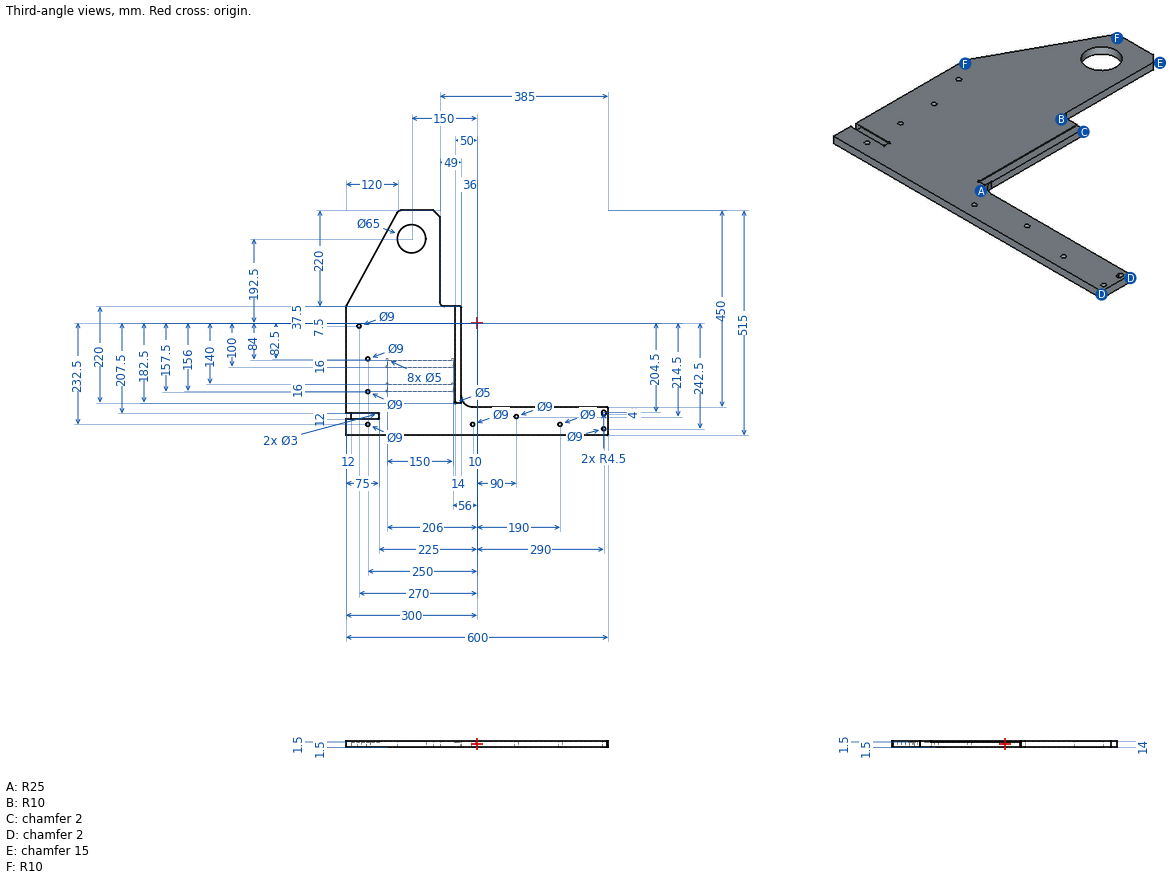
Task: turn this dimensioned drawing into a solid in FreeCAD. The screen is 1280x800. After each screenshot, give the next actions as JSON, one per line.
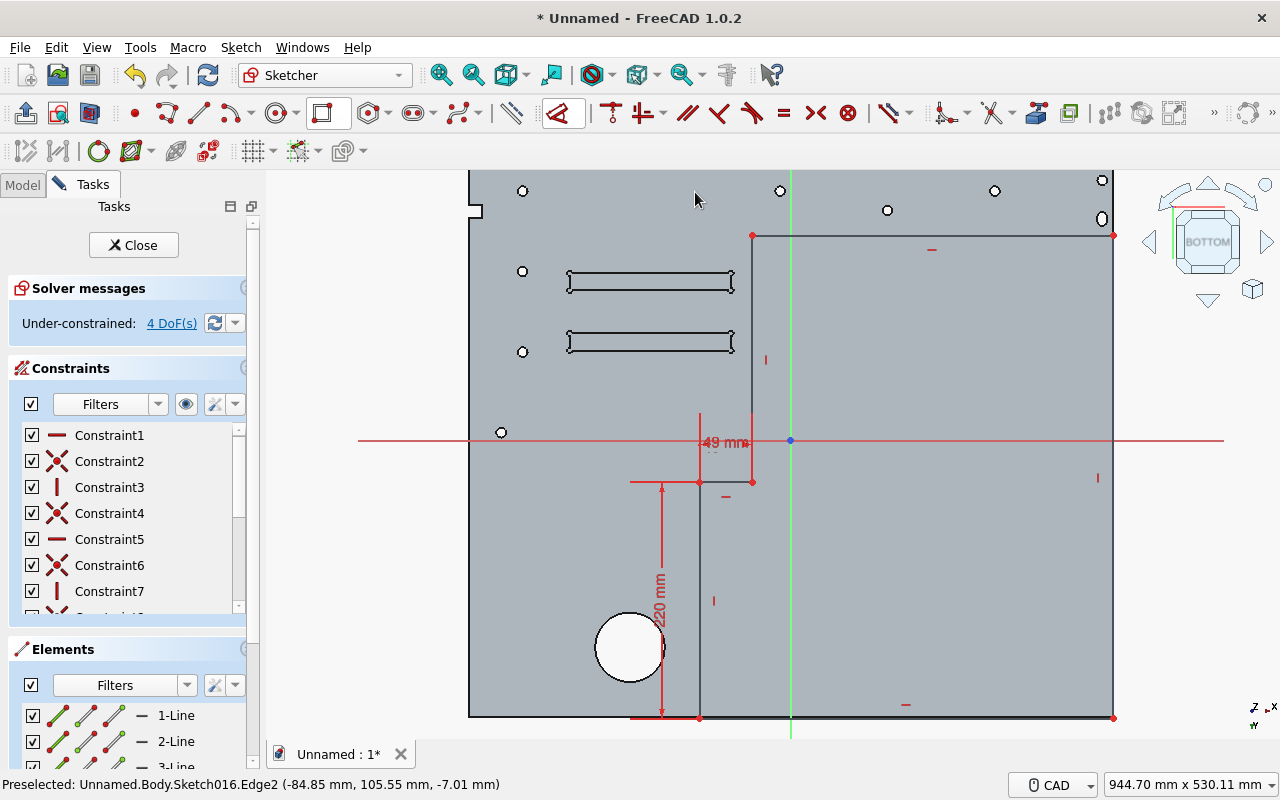
{"action": "scroll", "coordinate": [294, 359], "scroll_direction": "down", "scroll_amount": 1}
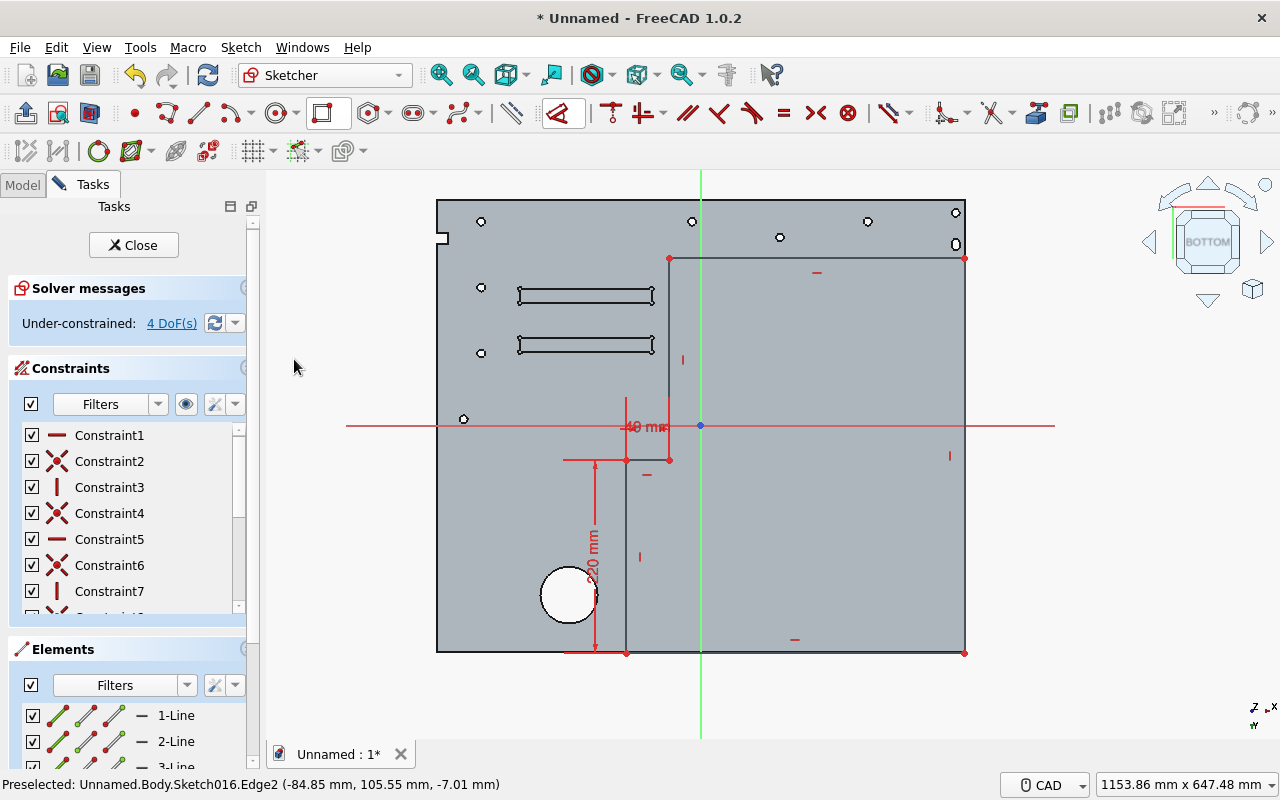
{"action": "left_click", "coordinate": [728, 653]}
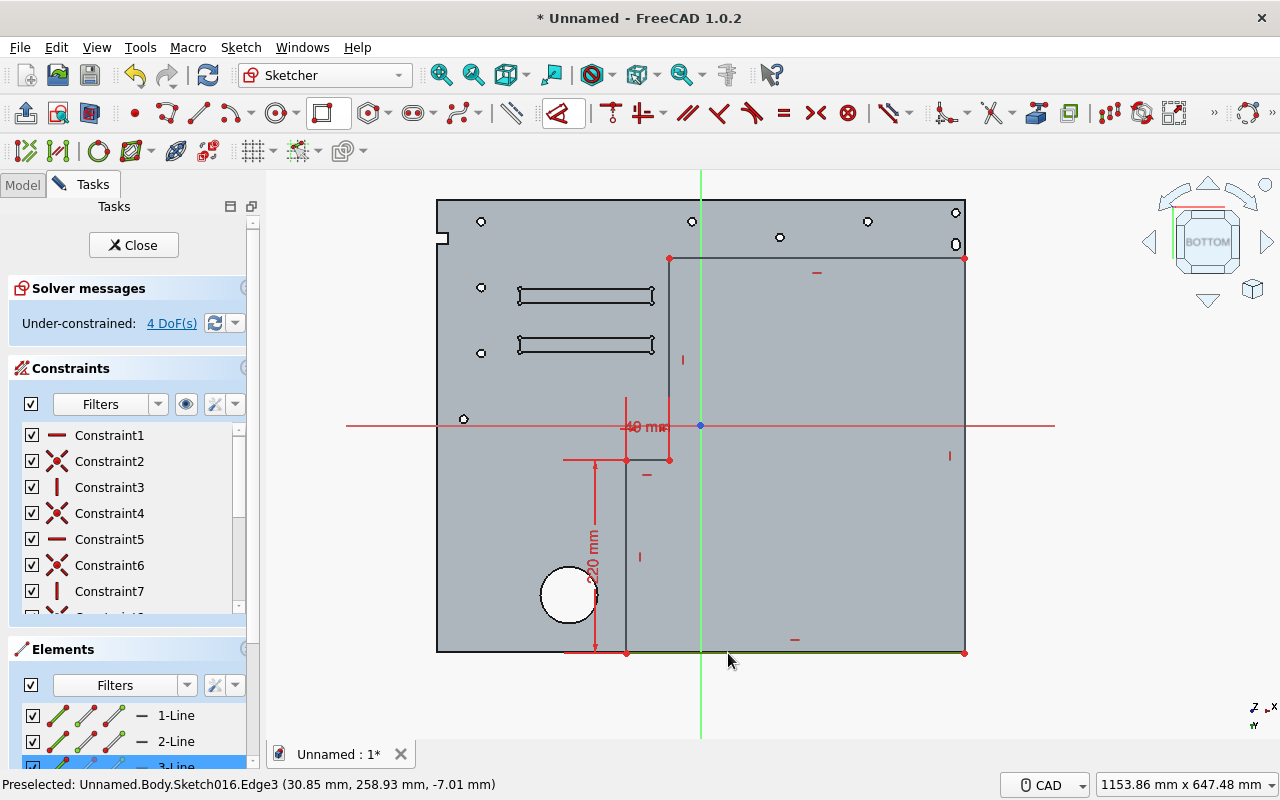
{"action": "left_click", "coordinate": [580, 114]}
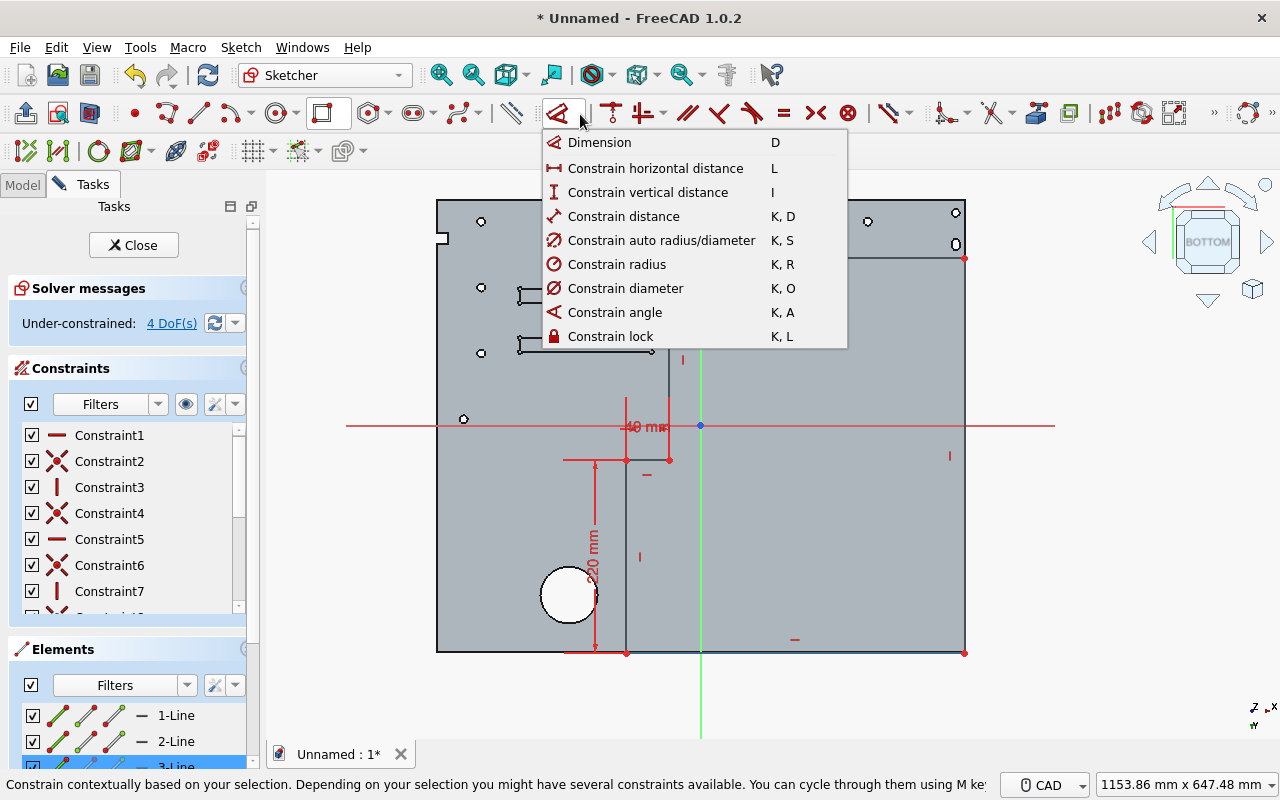
{"action": "left_click", "coordinate": [695, 168]}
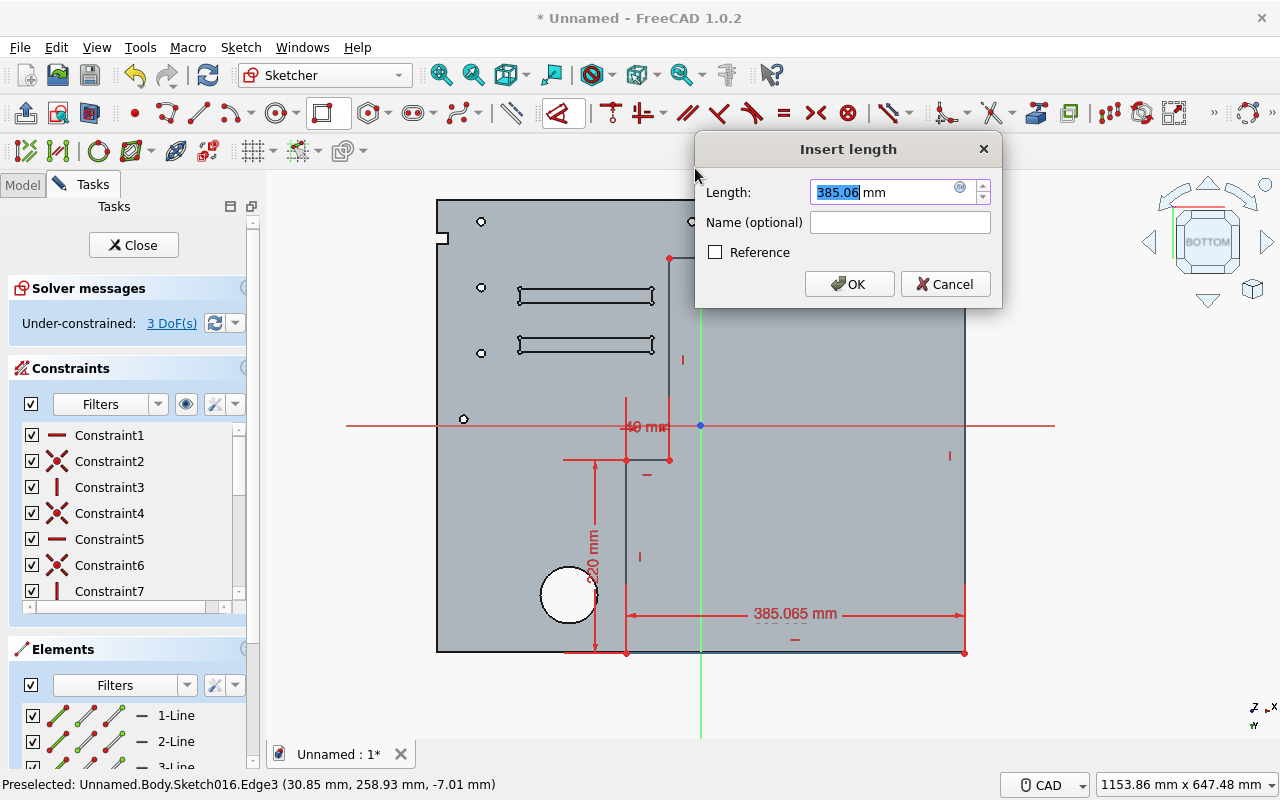
{"action": "type", "text": "385"}
{"action": "key", "text": "Return"}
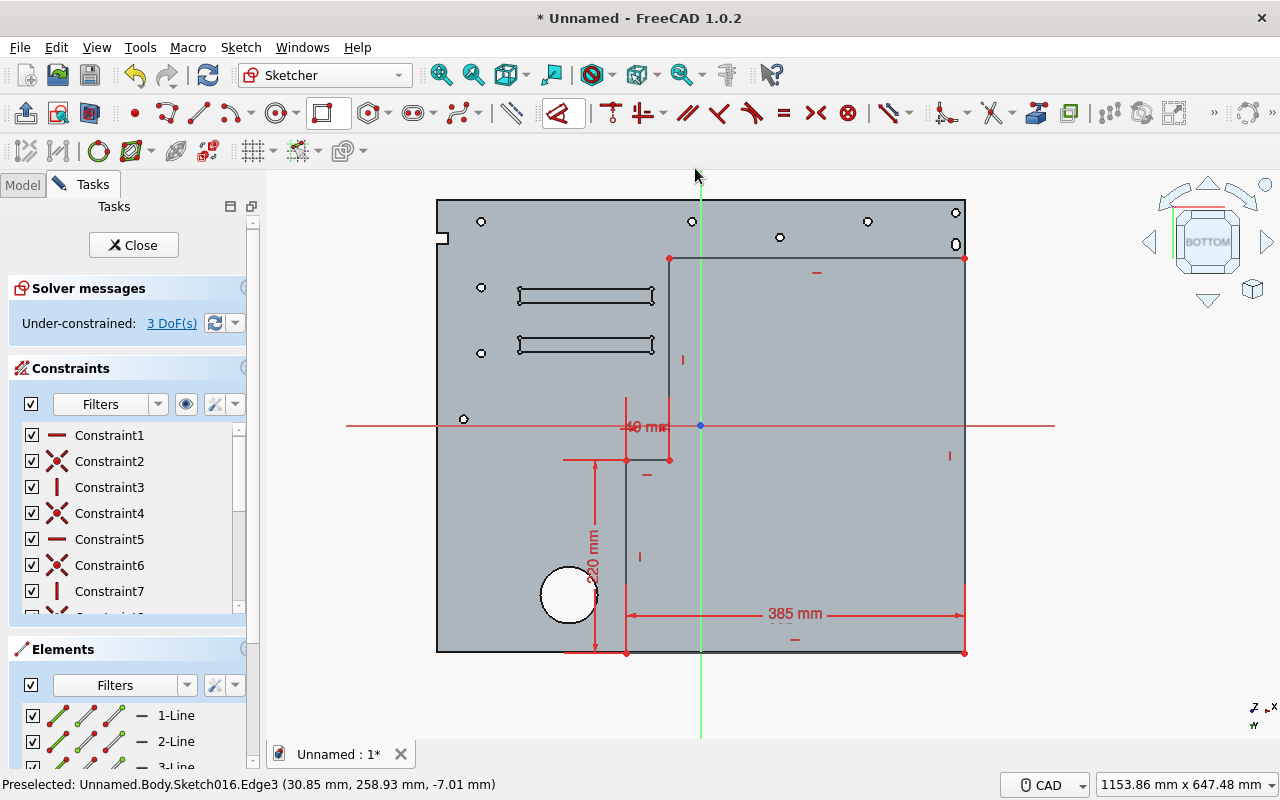
{"action": "left_click", "coordinate": [965, 535]}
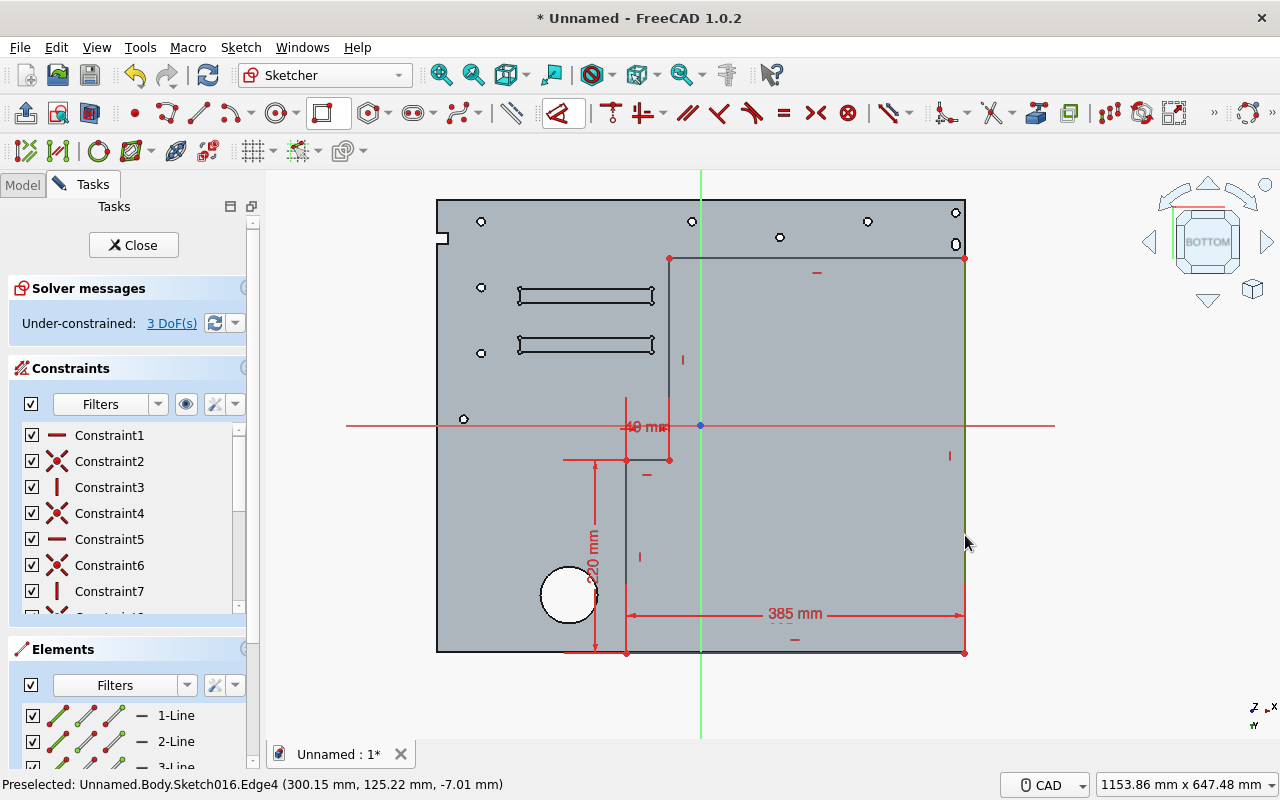
{"action": "left_click", "coordinate": [580, 114]}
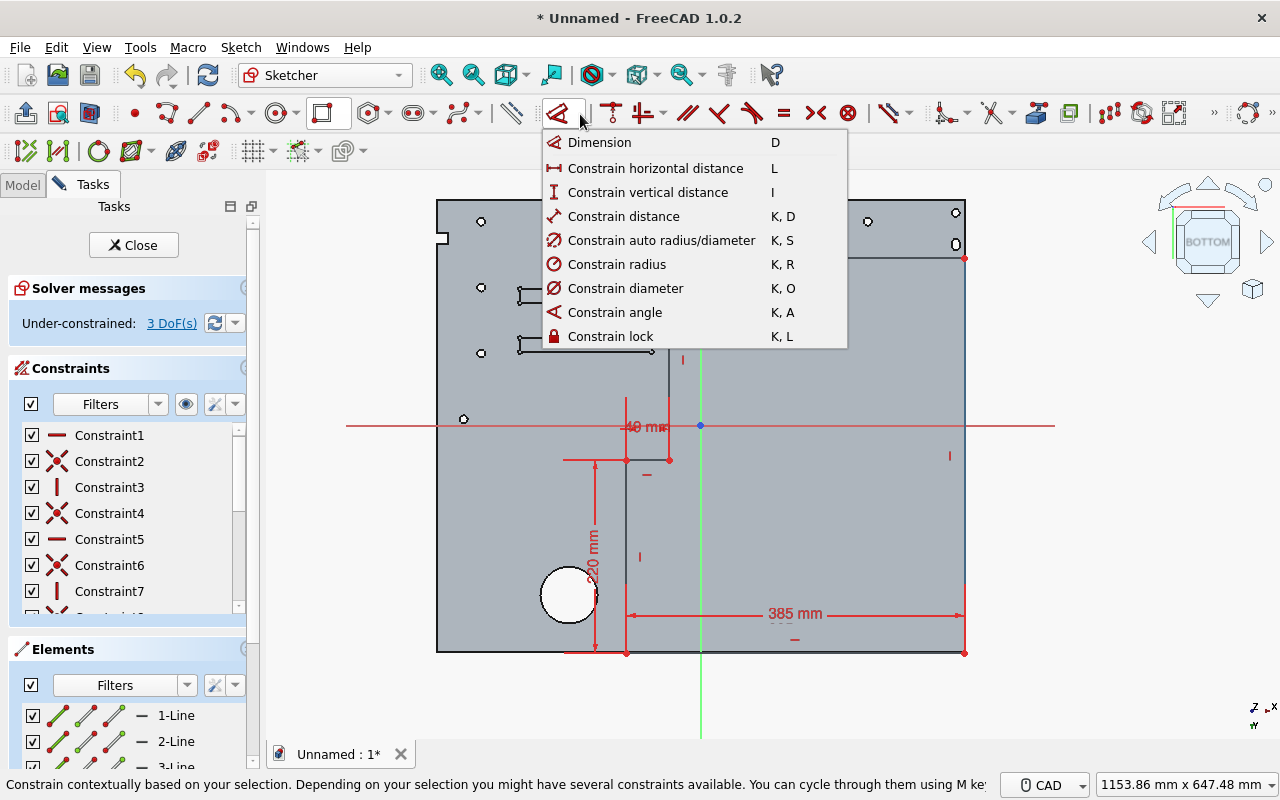
{"action": "left_click", "coordinate": [695, 192]}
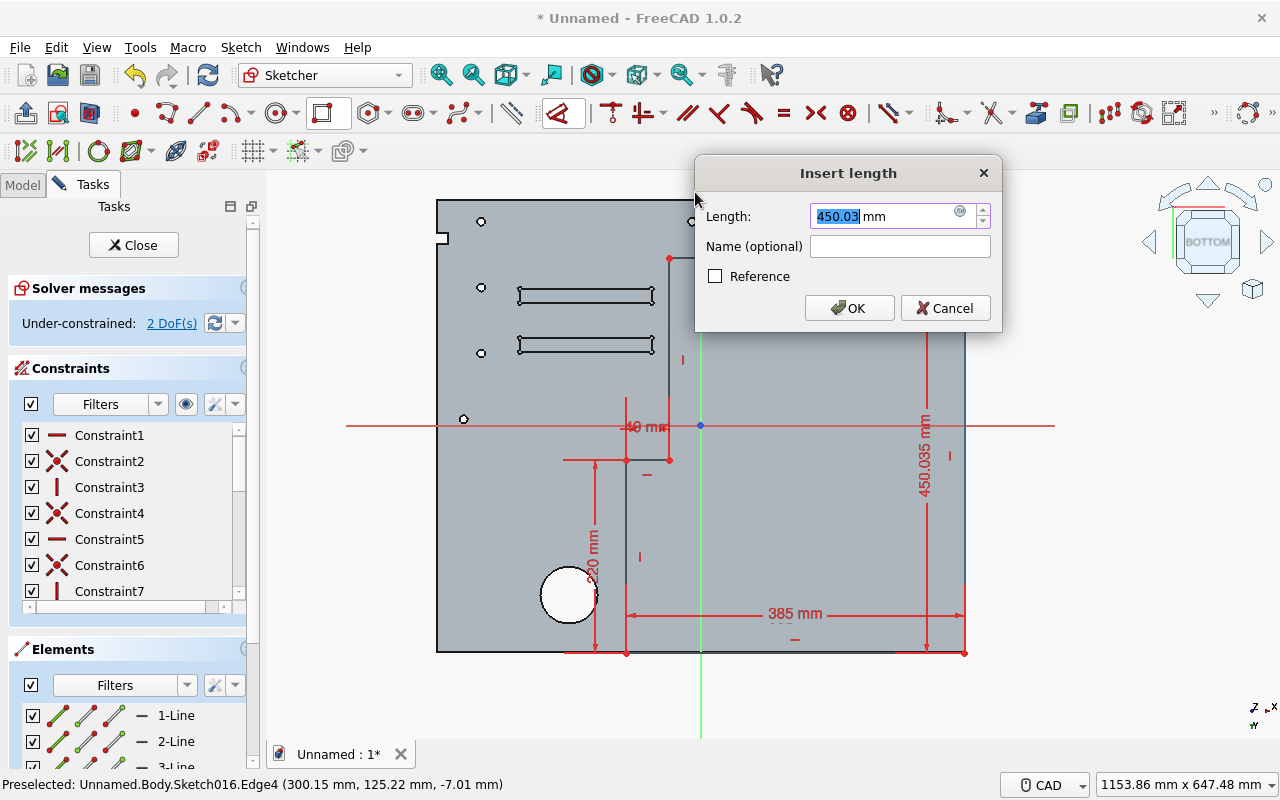
{"action": "type", "text": "450"}
{"action": "key", "text": "Return"}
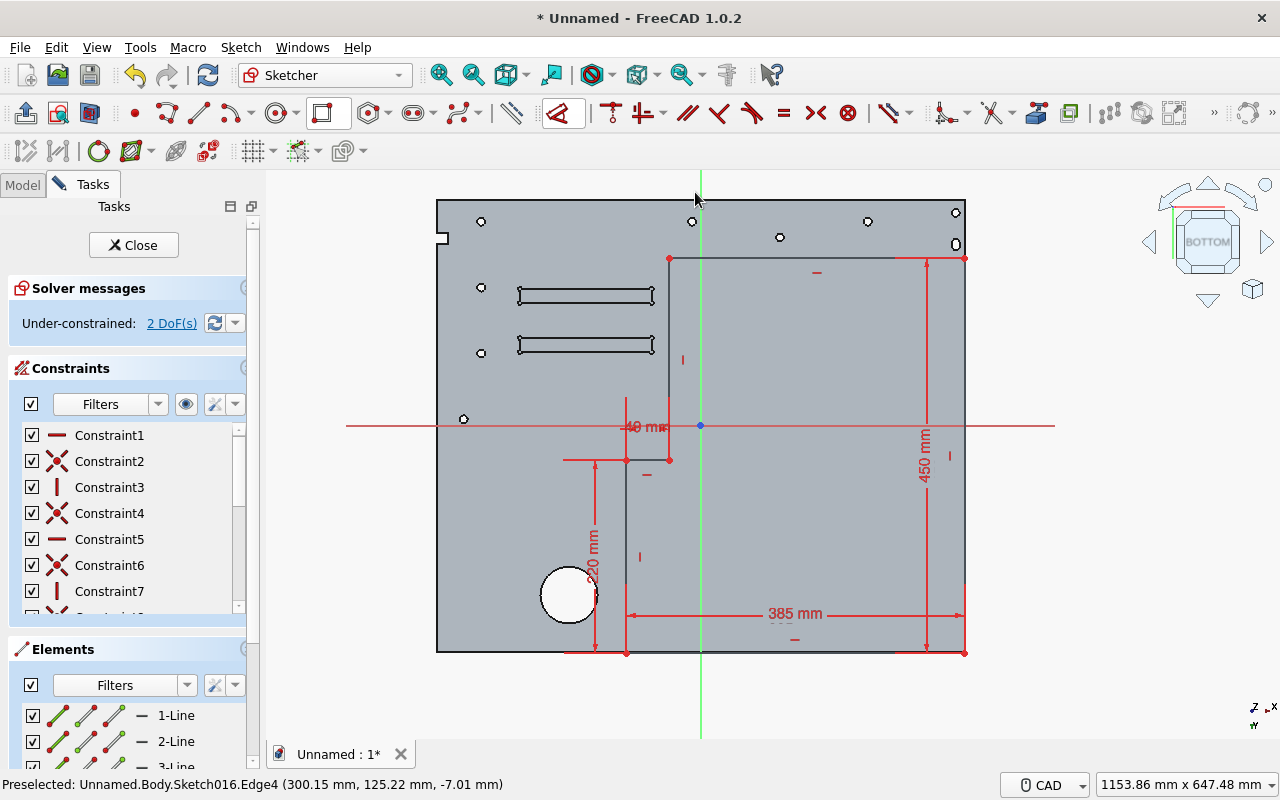
{"action": "scroll", "coordinate": [669, 460], "scroll_direction": "up", "scroll_amount": 2}